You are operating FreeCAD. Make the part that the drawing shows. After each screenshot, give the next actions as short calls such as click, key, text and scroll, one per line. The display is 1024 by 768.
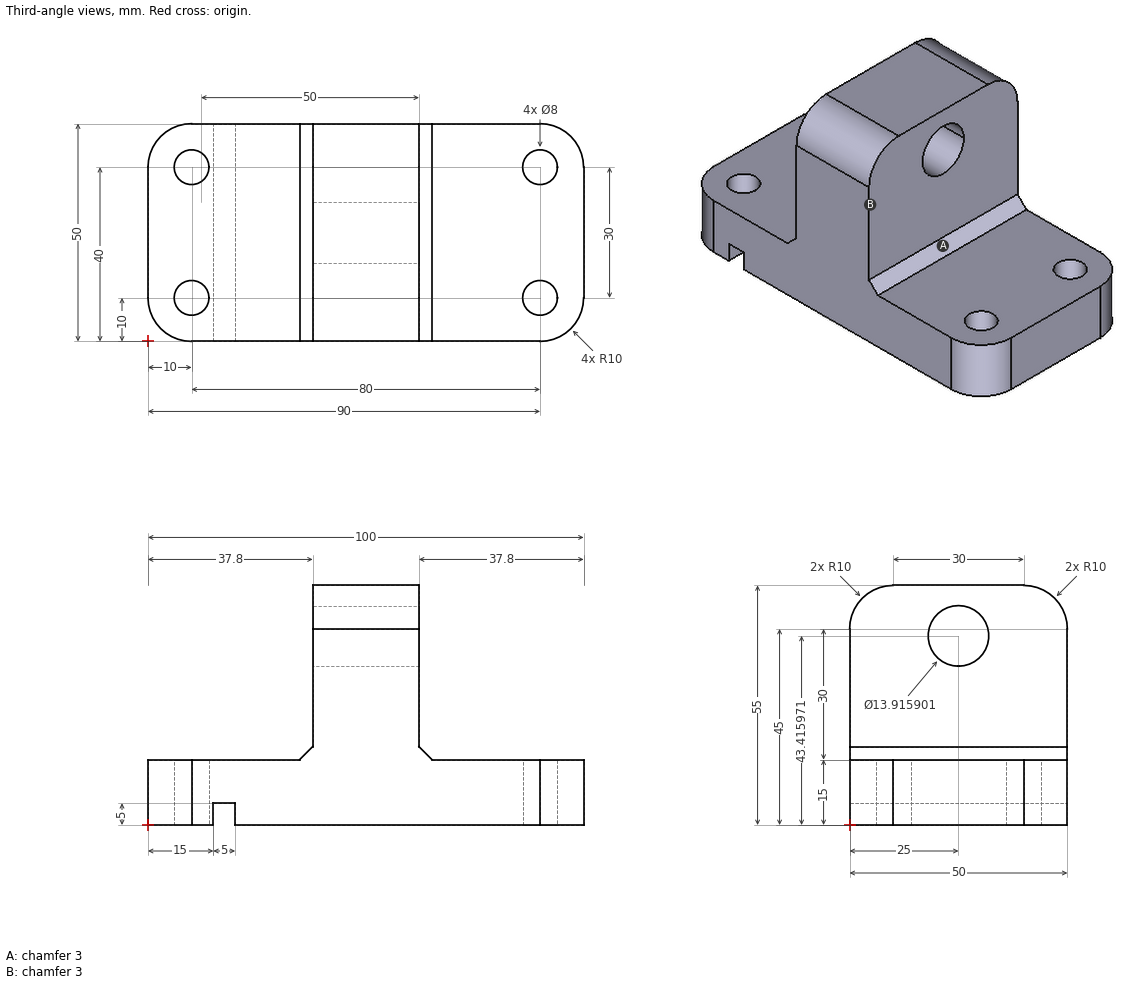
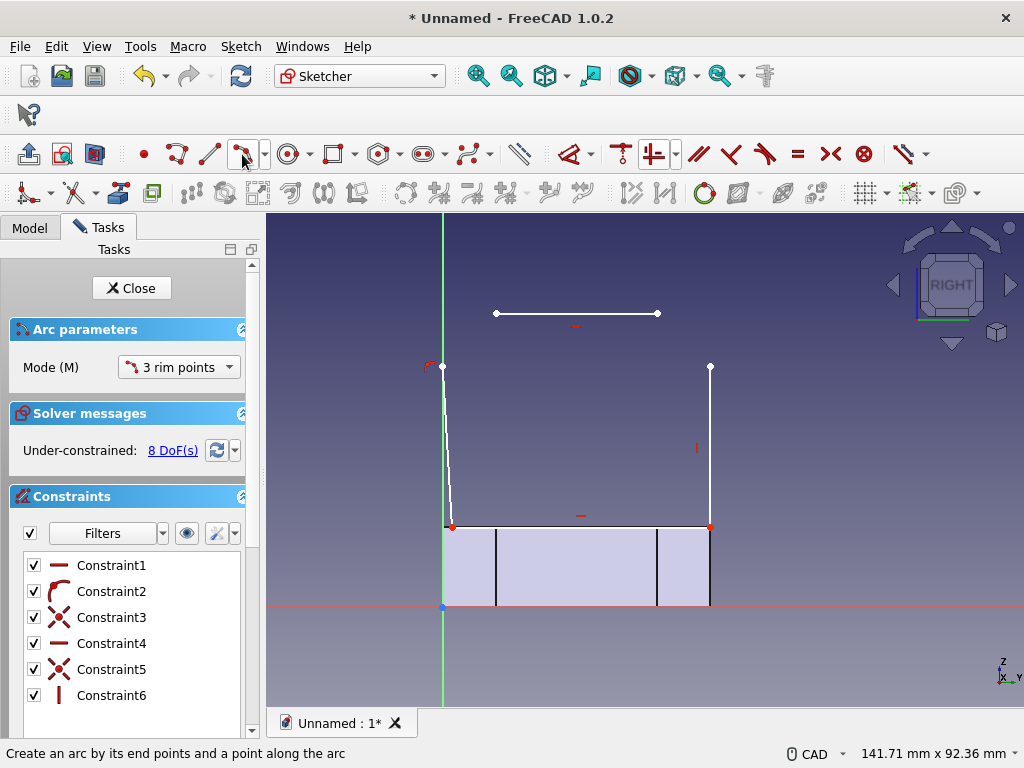
click(496, 314)
click(443, 367)
click(458, 329)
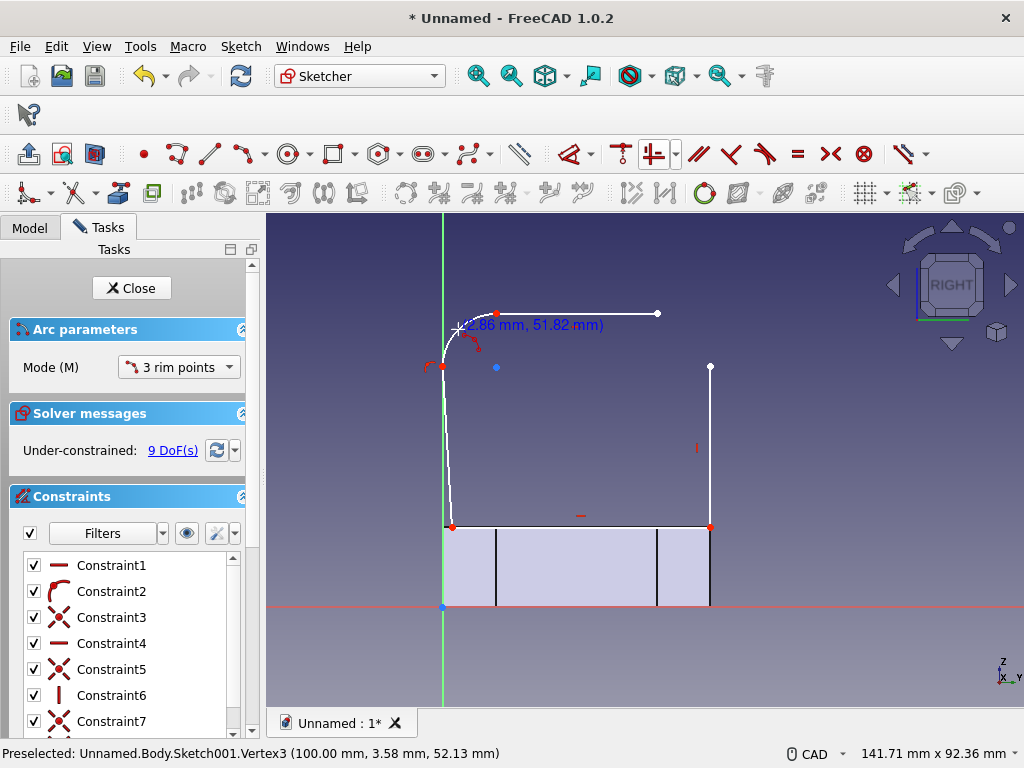
click(710, 367)
click(657, 314)
click(694, 329)
key(Escape)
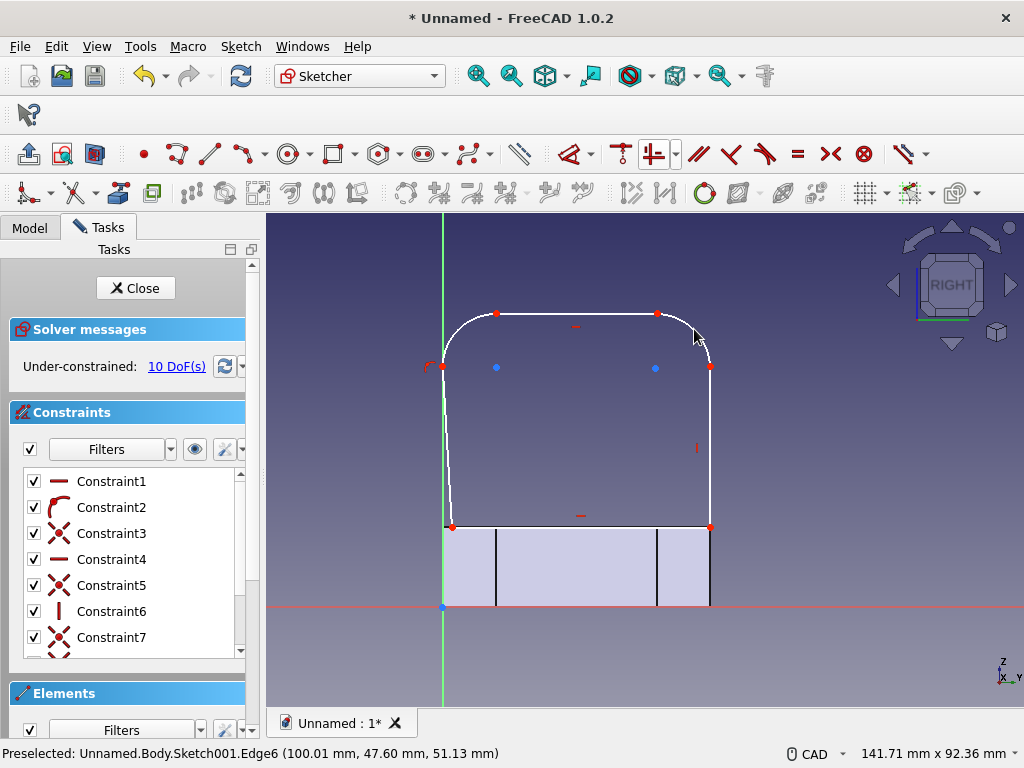
click(609, 314)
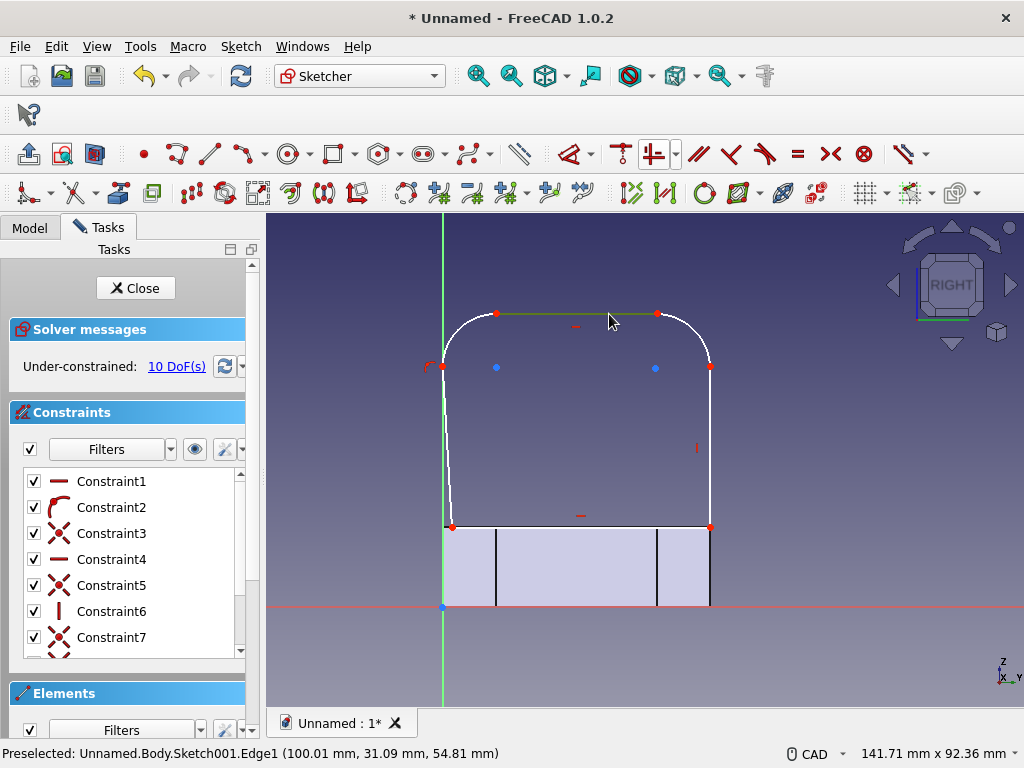
click(472, 320)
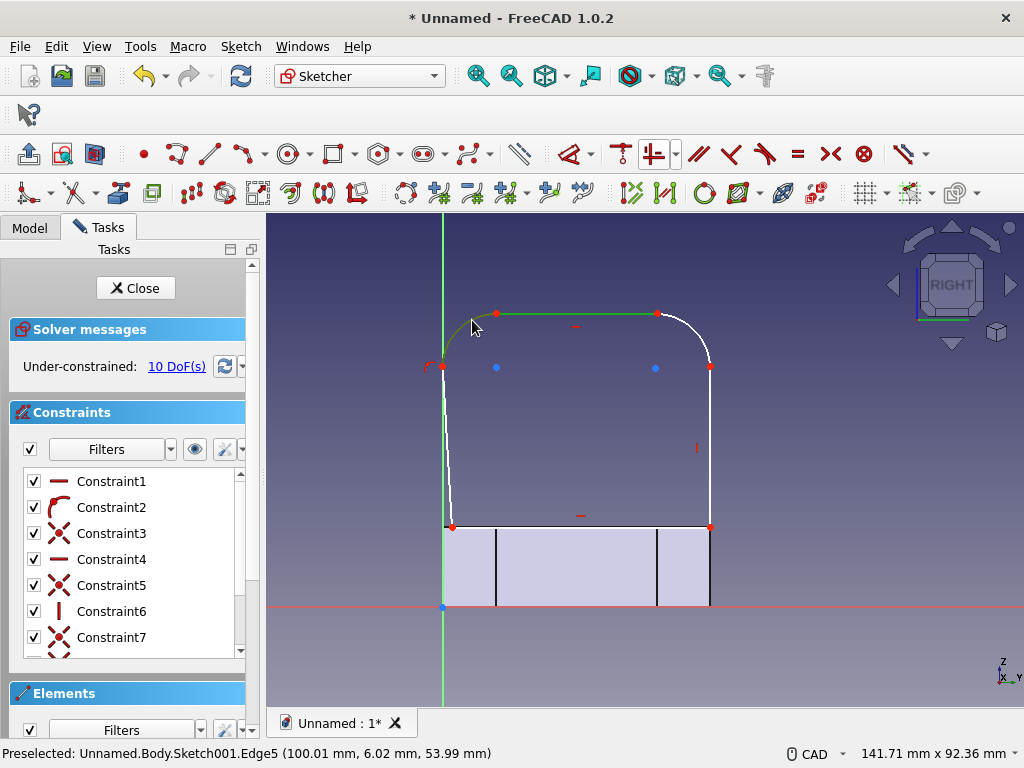
click(765, 154)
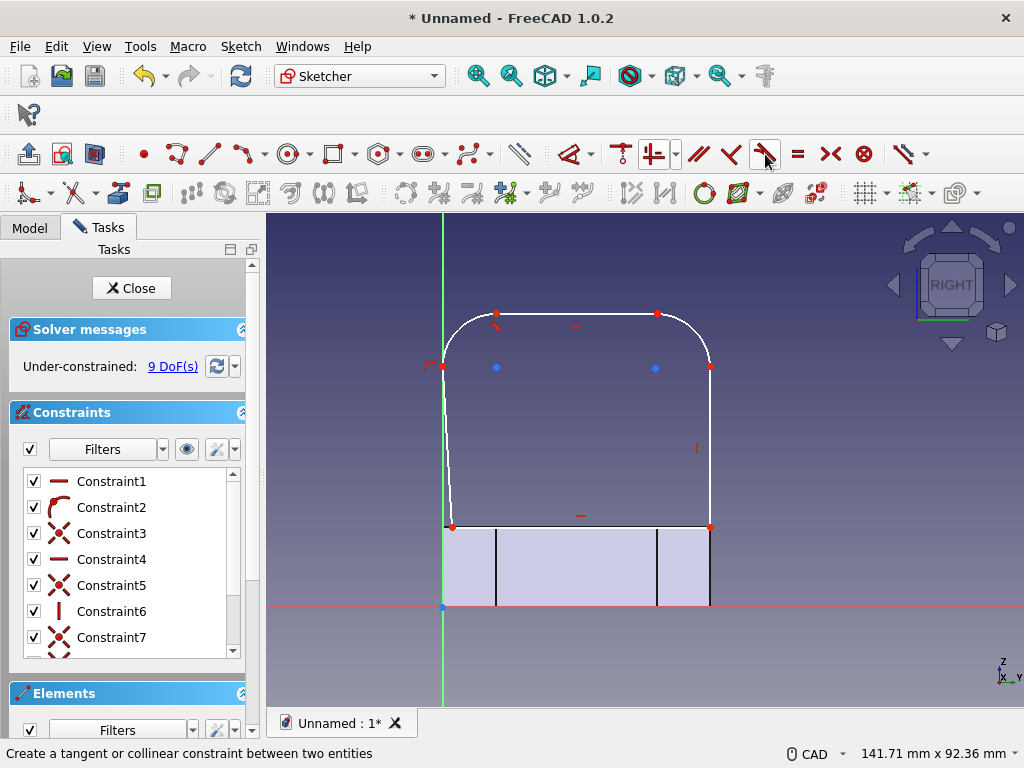
click(609, 314)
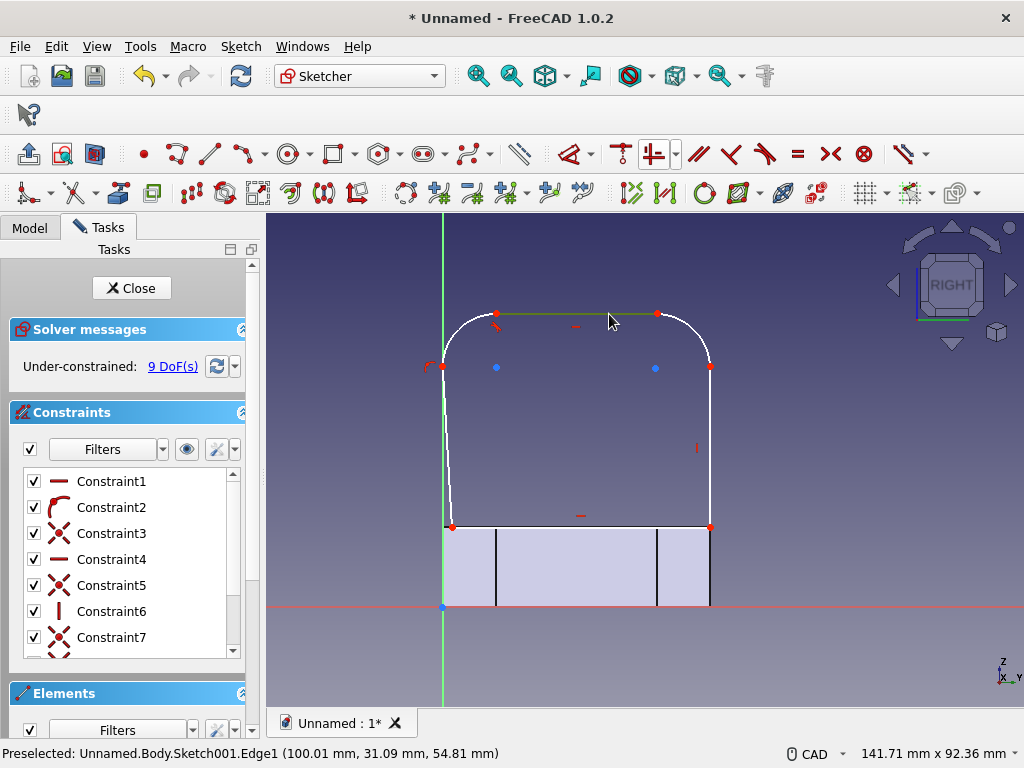
click(704, 343)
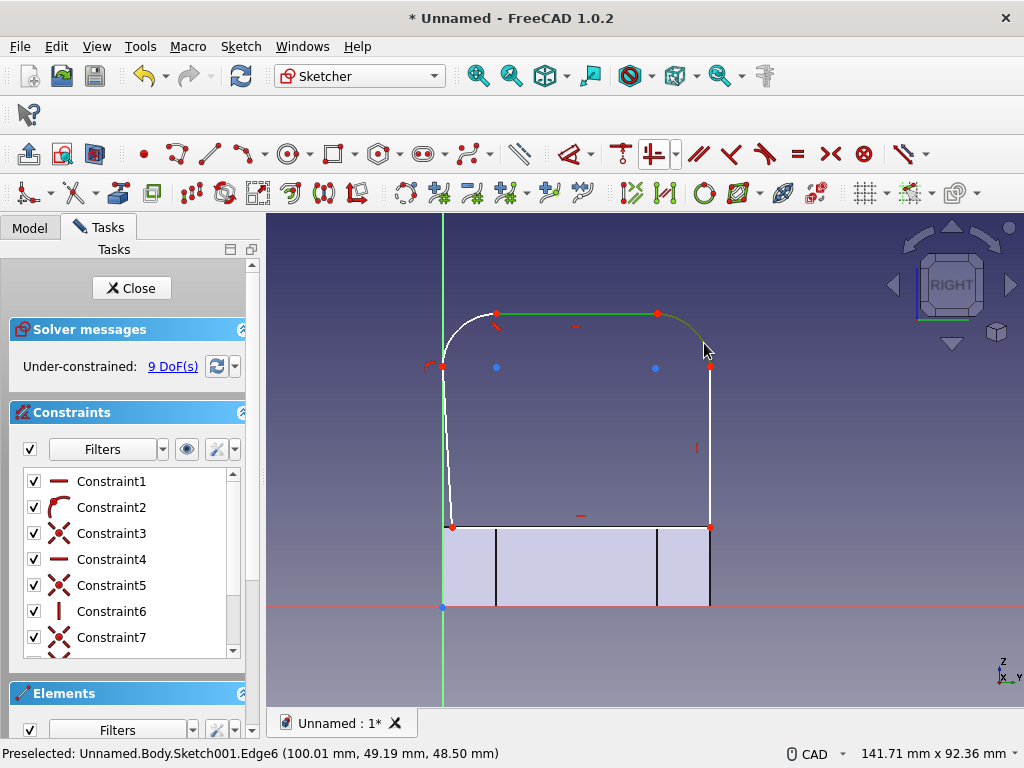
click(765, 154)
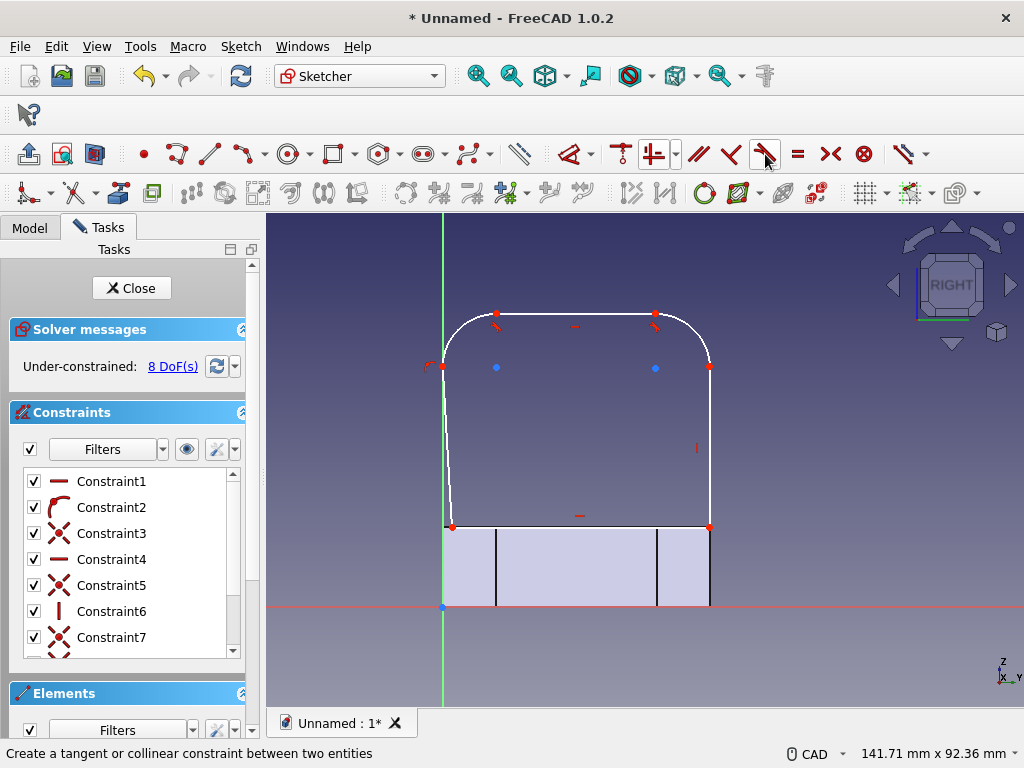
click(446, 415)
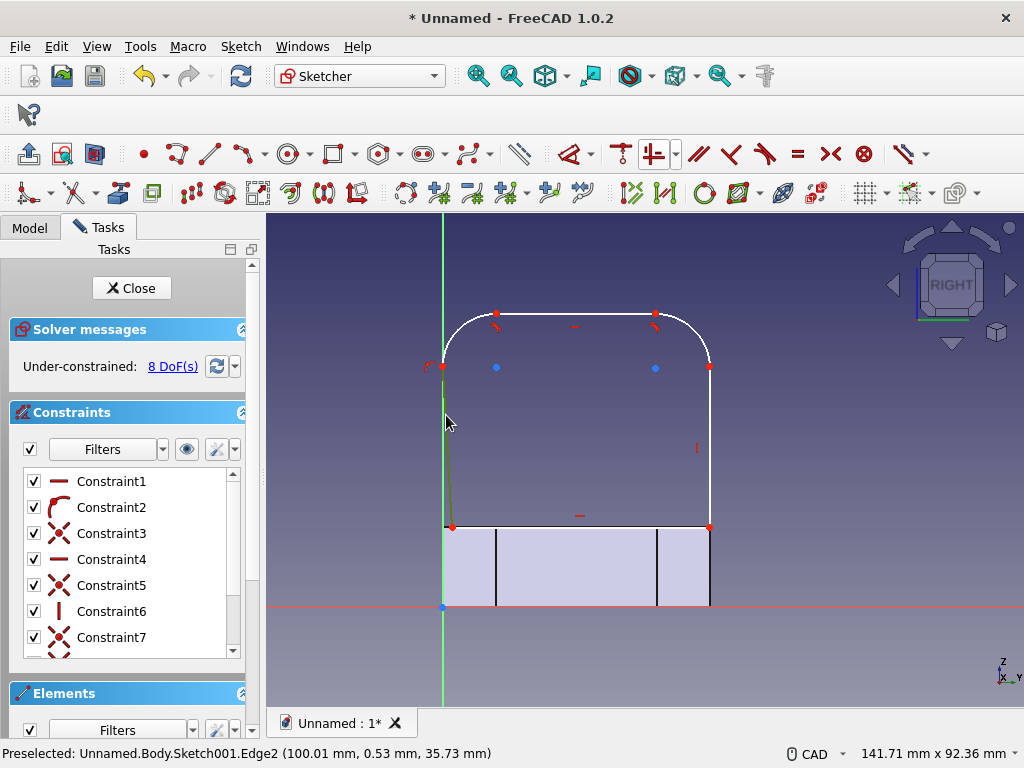
click(472, 320)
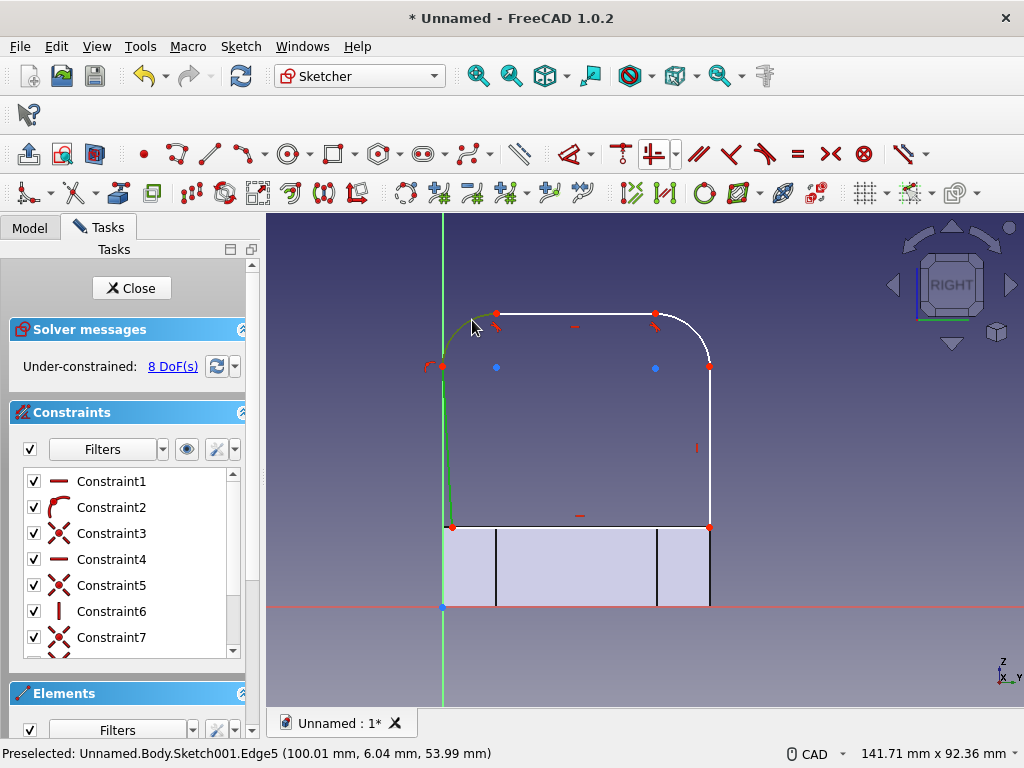
click(765, 154)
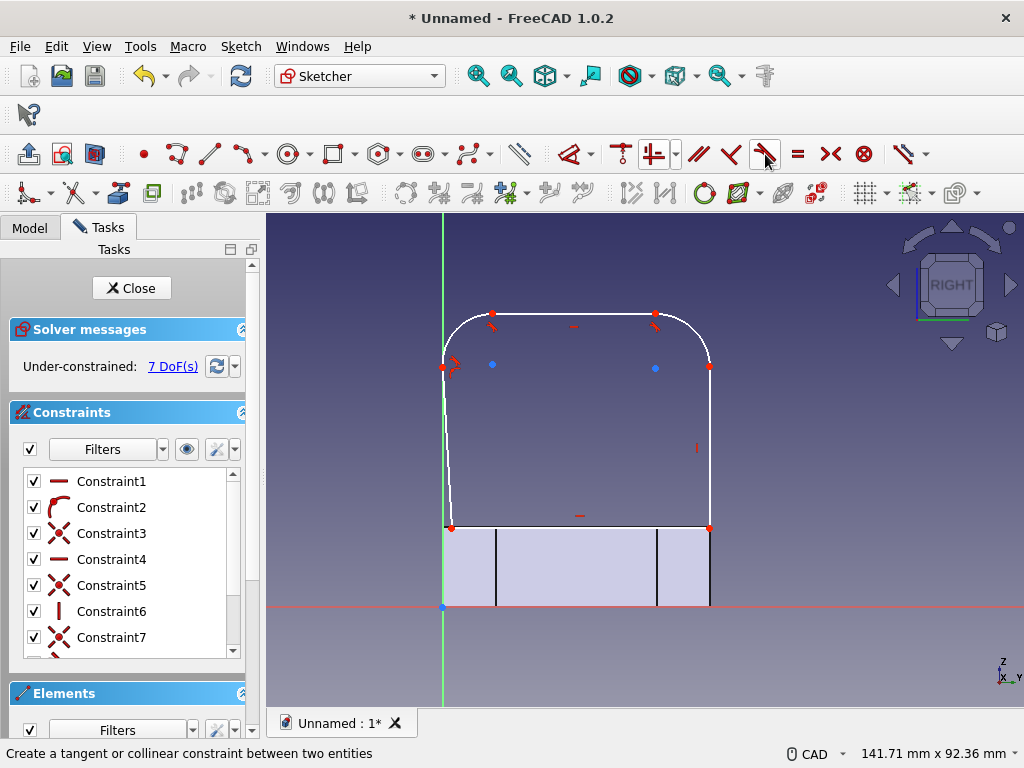
click(710, 480)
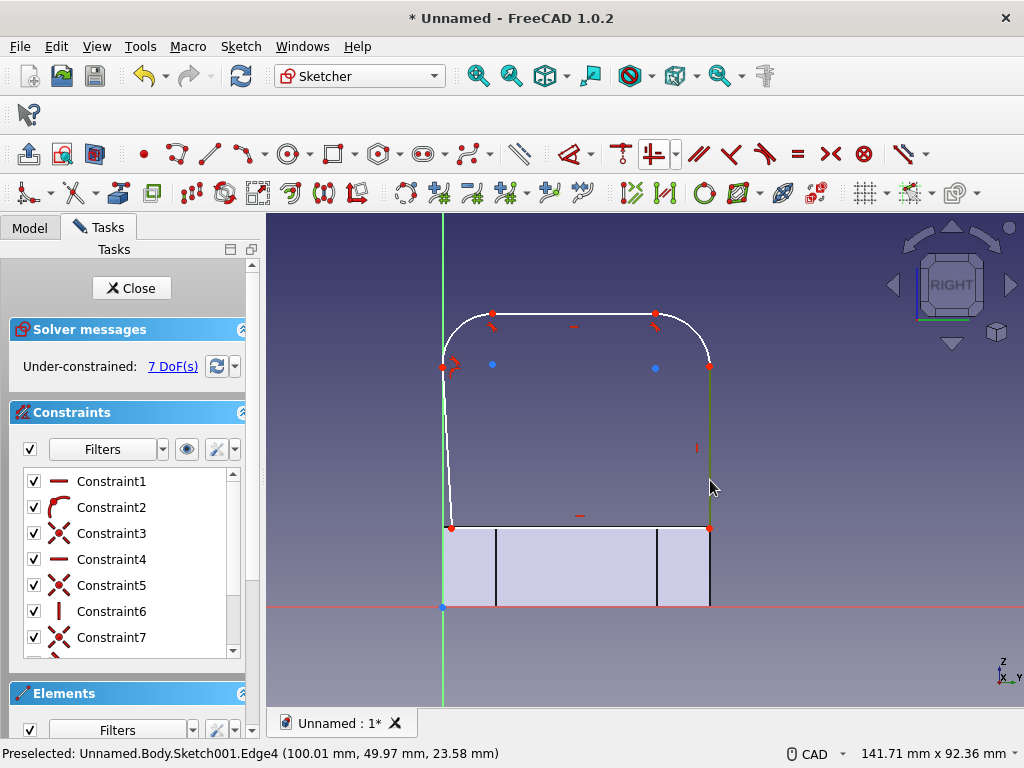
click(703, 343)